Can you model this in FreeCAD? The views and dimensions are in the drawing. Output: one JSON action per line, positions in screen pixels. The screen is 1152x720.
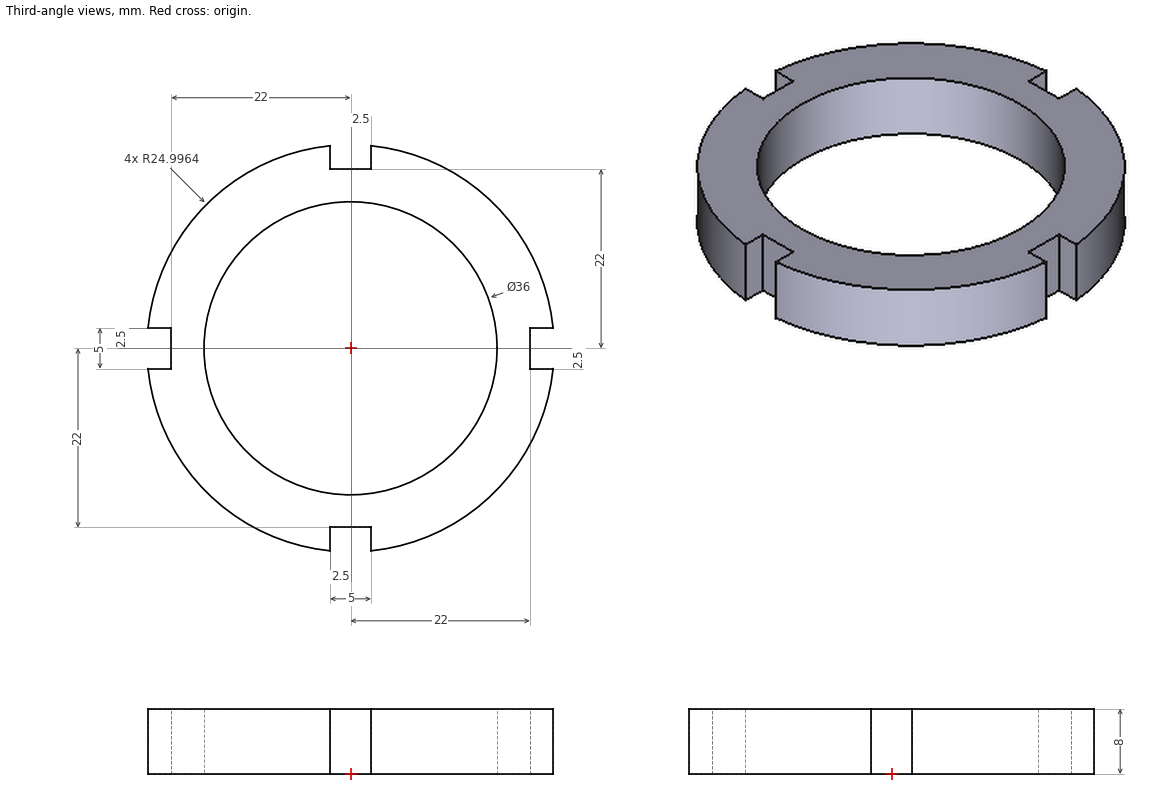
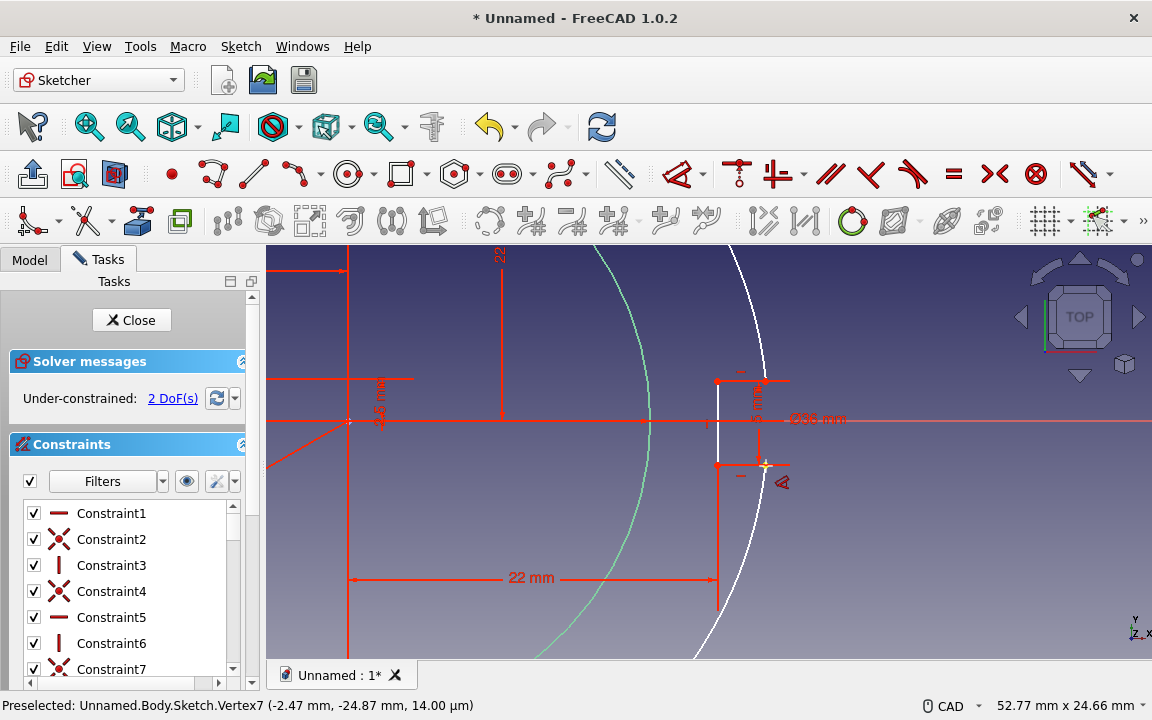
{"action": "left_click", "coordinate": [765, 465]}
{"action": "left_click", "coordinate": [799, 443]}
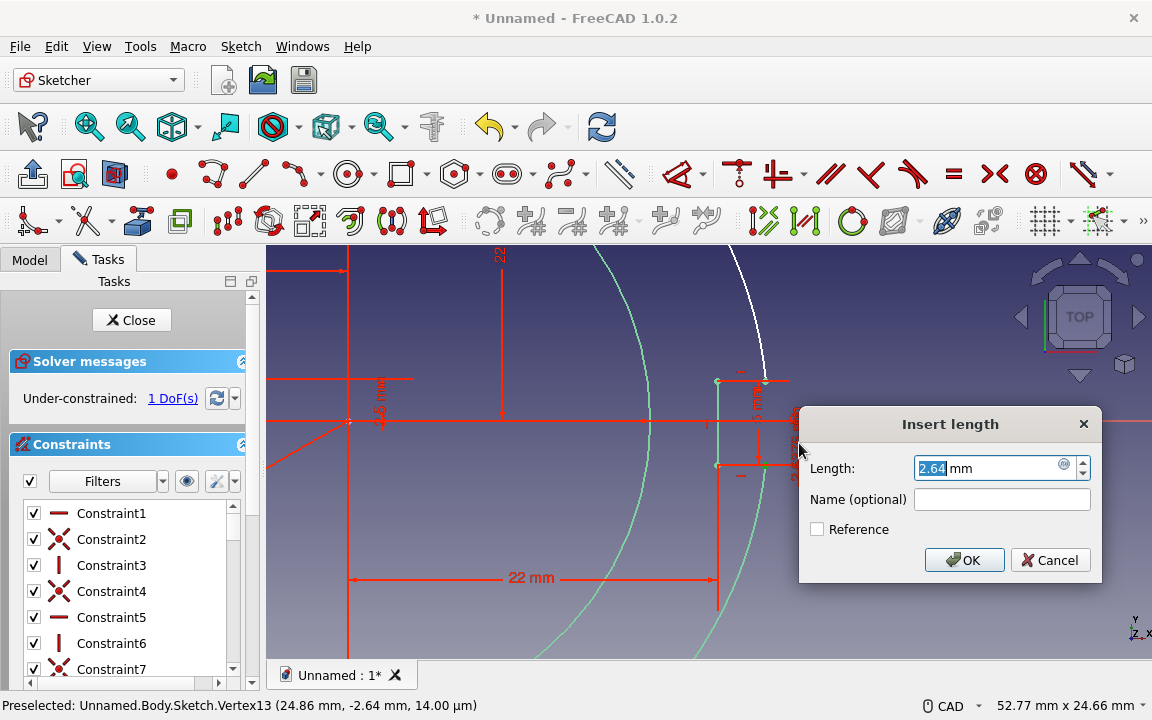
{"action": "type", "text": "2.5"}
{"action": "key", "text": "Return"}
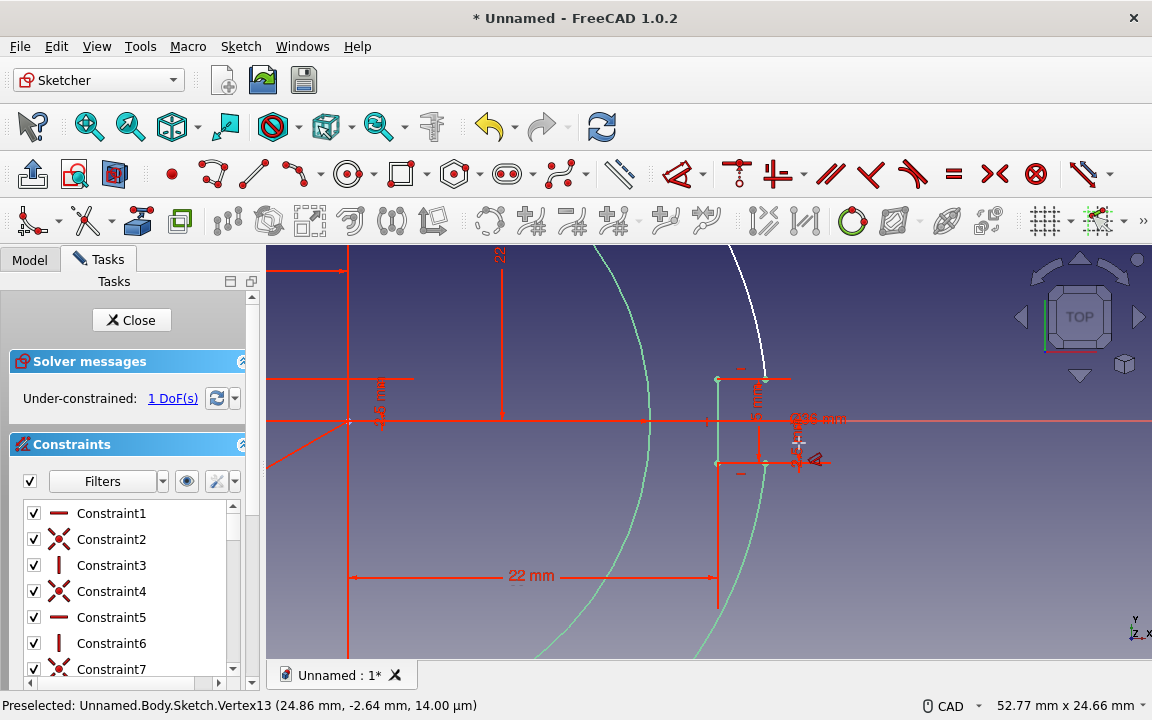
{"action": "scroll", "coordinate": [767, 465], "scroll_direction": "down", "scroll_amount": 6}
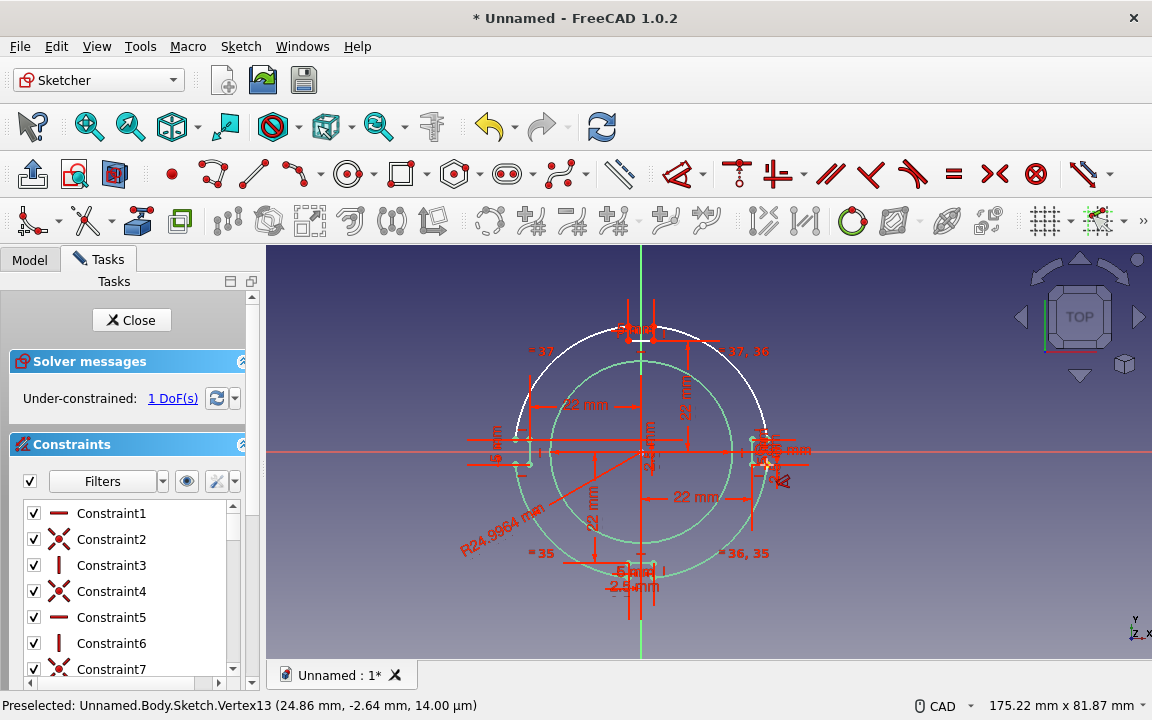
{"action": "scroll", "coordinate": [654, 326], "scroll_direction": "up", "scroll_amount": 6}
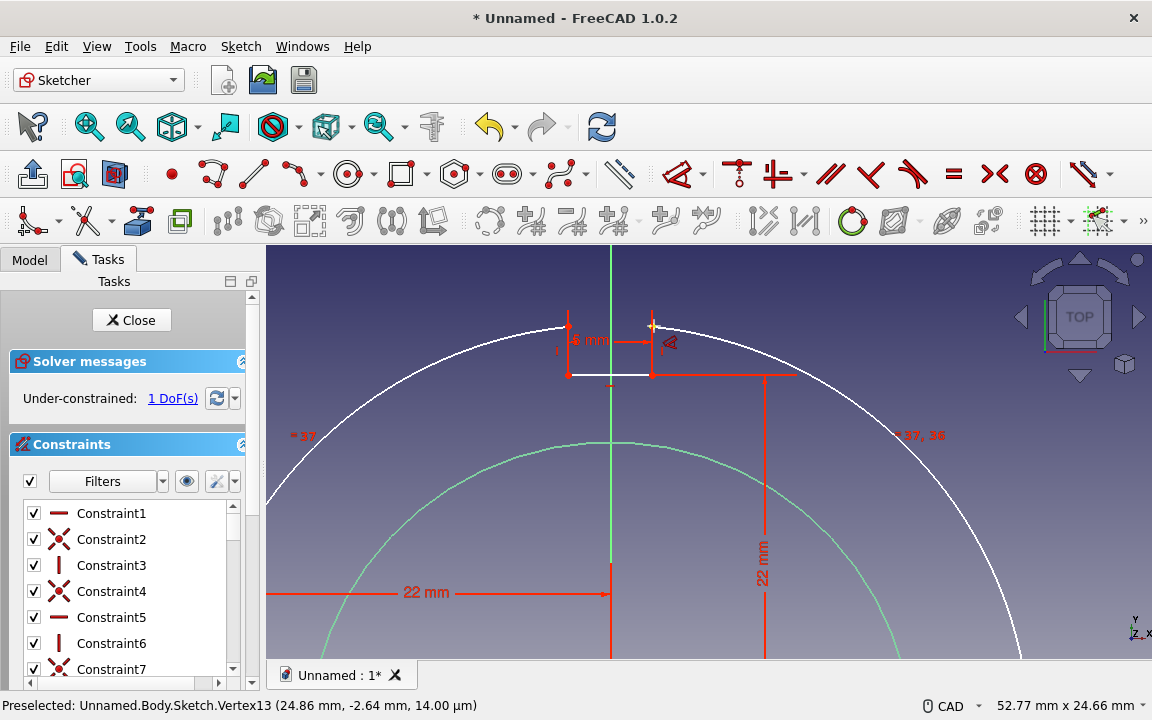
{"action": "left_click", "coordinate": [652, 327]}
{"action": "left_click", "coordinate": [631, 293]}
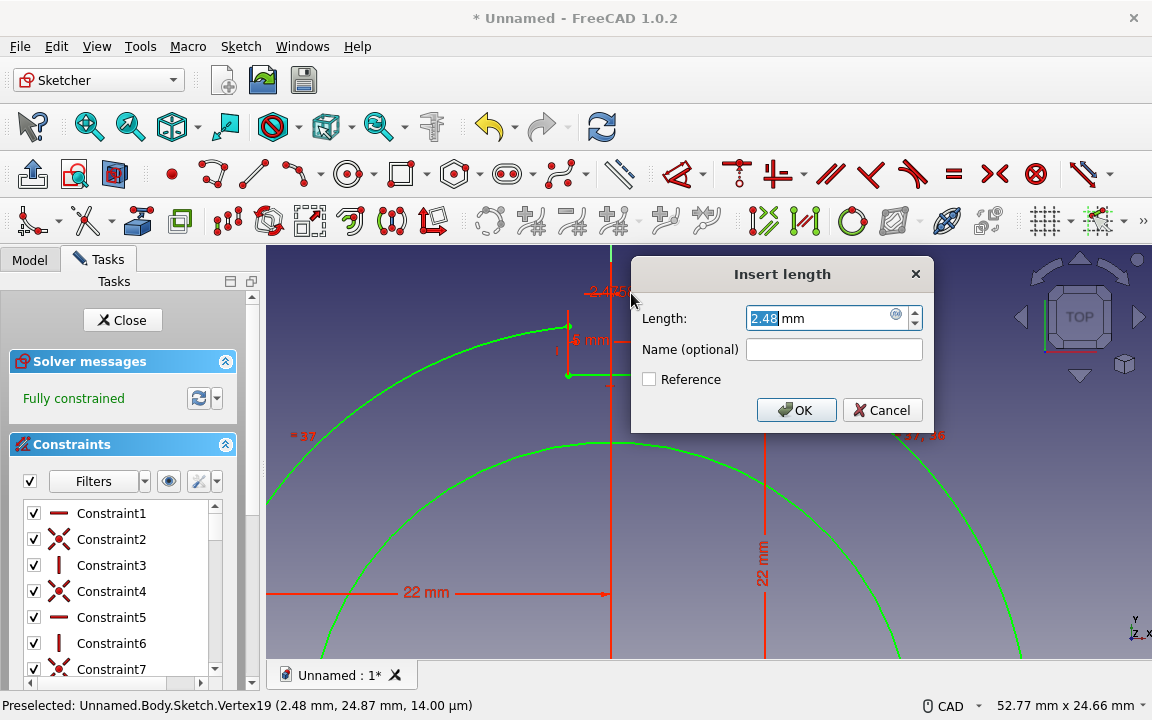
{"action": "type", "text": "2.5"}
{"action": "key", "text": "Return"}
{"action": "key", "text": "Escape"}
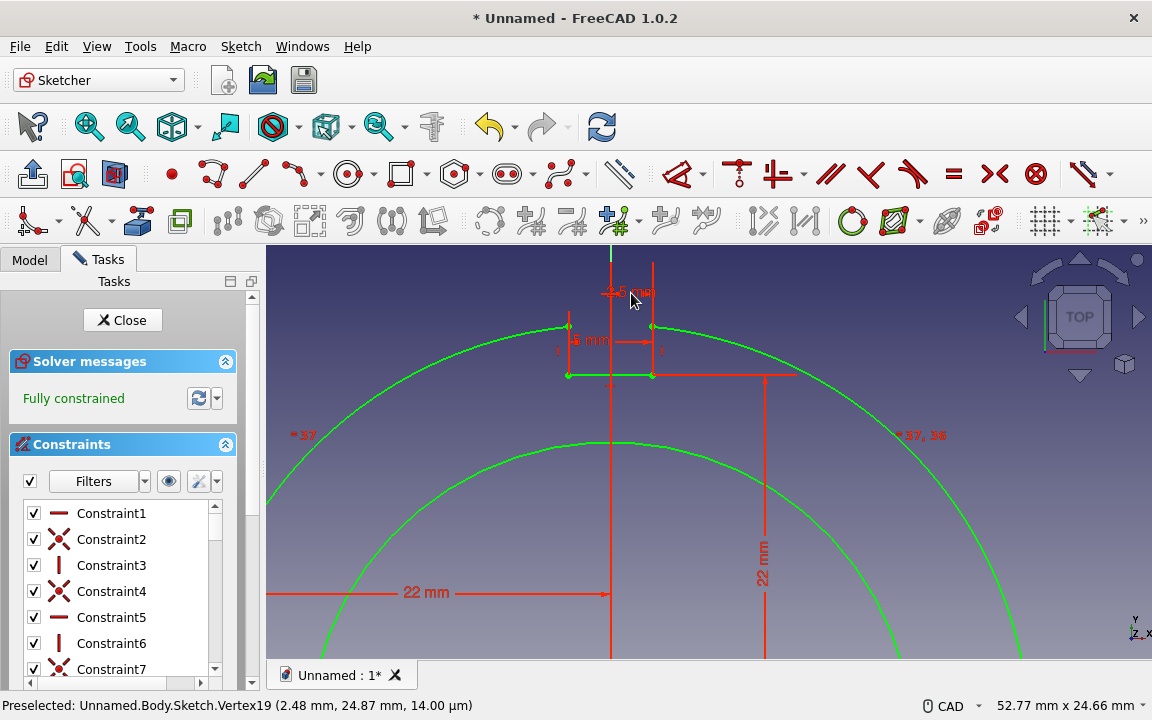
{"action": "left_click", "coordinate": [123, 320]}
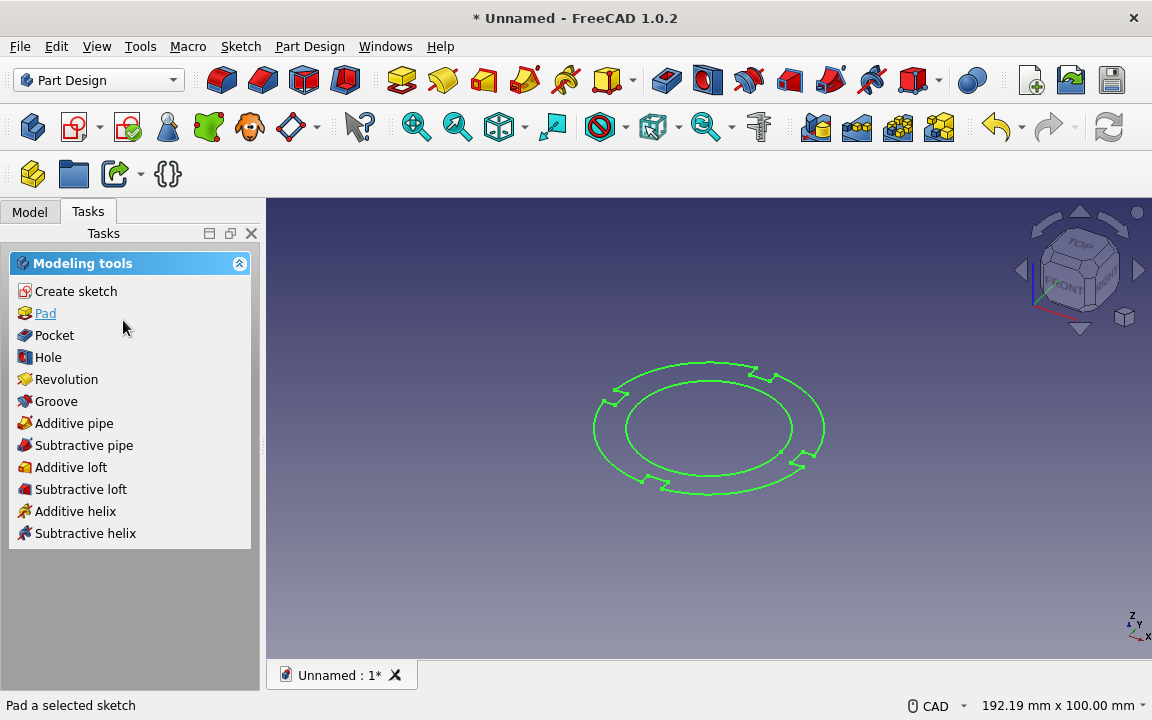
{"action": "left_click", "coordinate": [402, 80]}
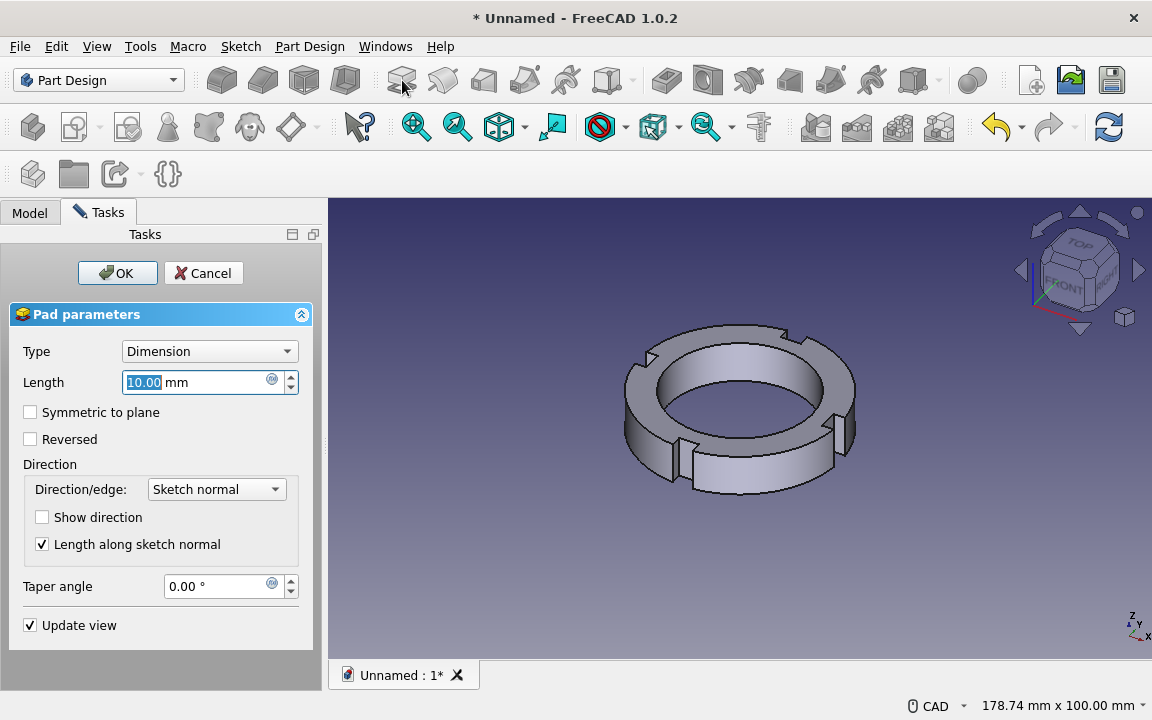
{"action": "type", "text": "8"}
{"action": "key", "text": "Tab"}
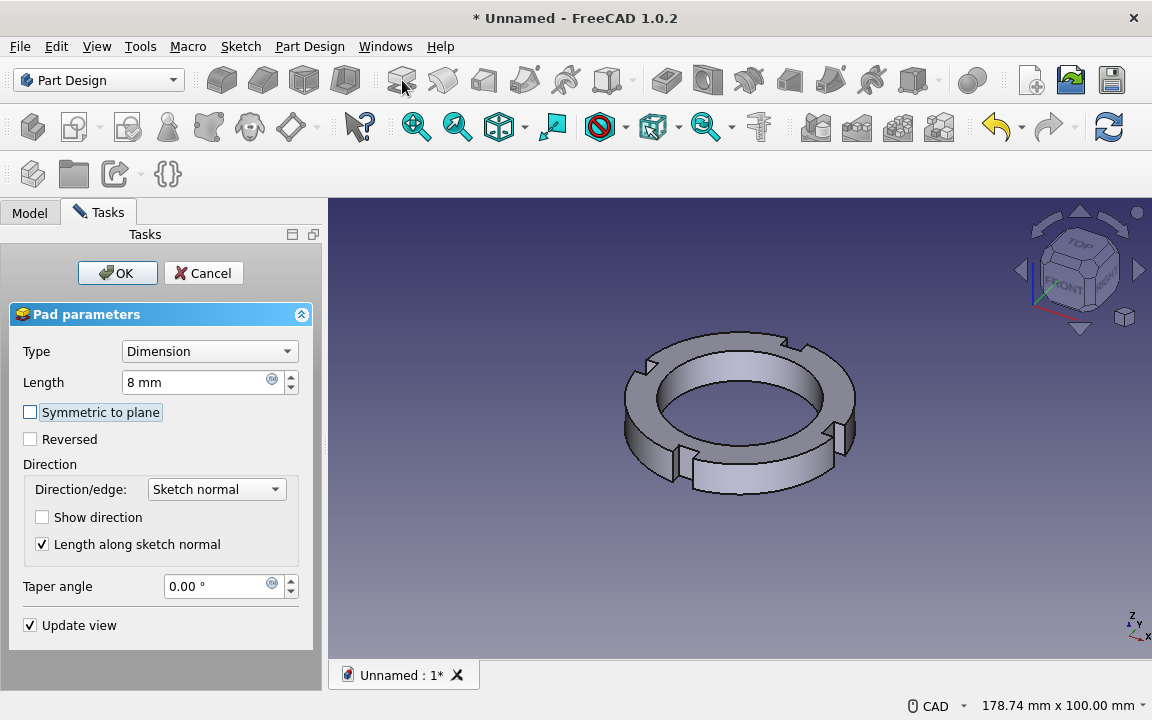
{"action": "left_click", "coordinate": [118, 273]}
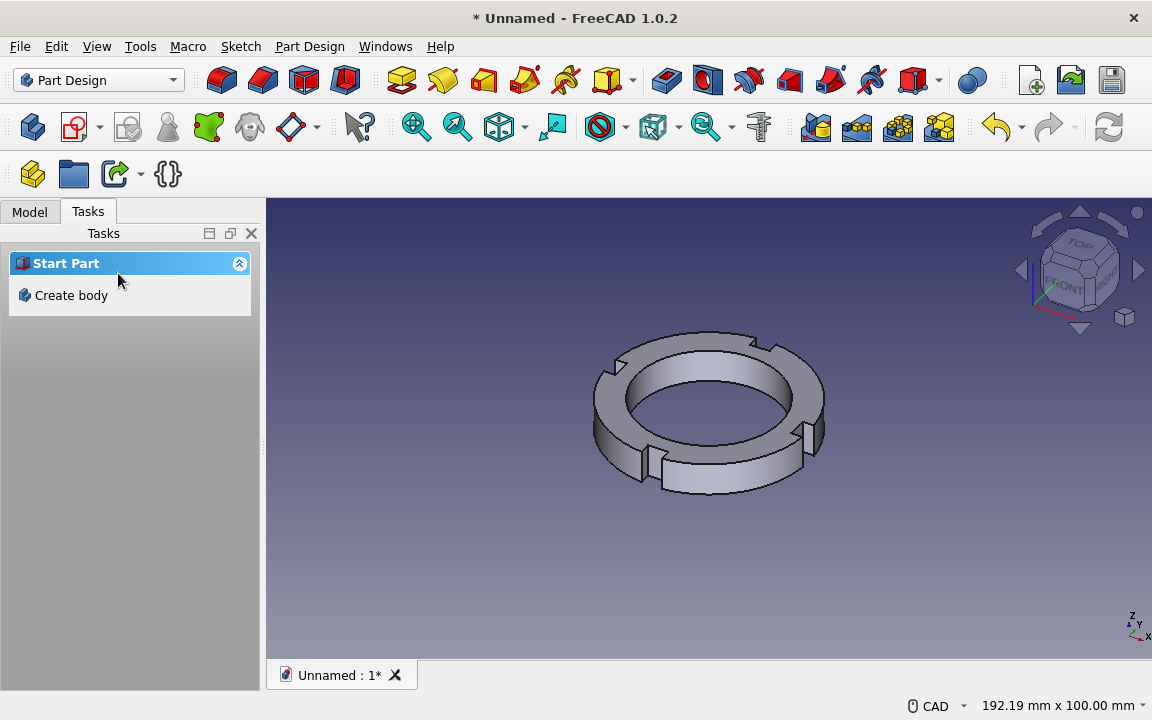
{"action": "key", "text": "0"}